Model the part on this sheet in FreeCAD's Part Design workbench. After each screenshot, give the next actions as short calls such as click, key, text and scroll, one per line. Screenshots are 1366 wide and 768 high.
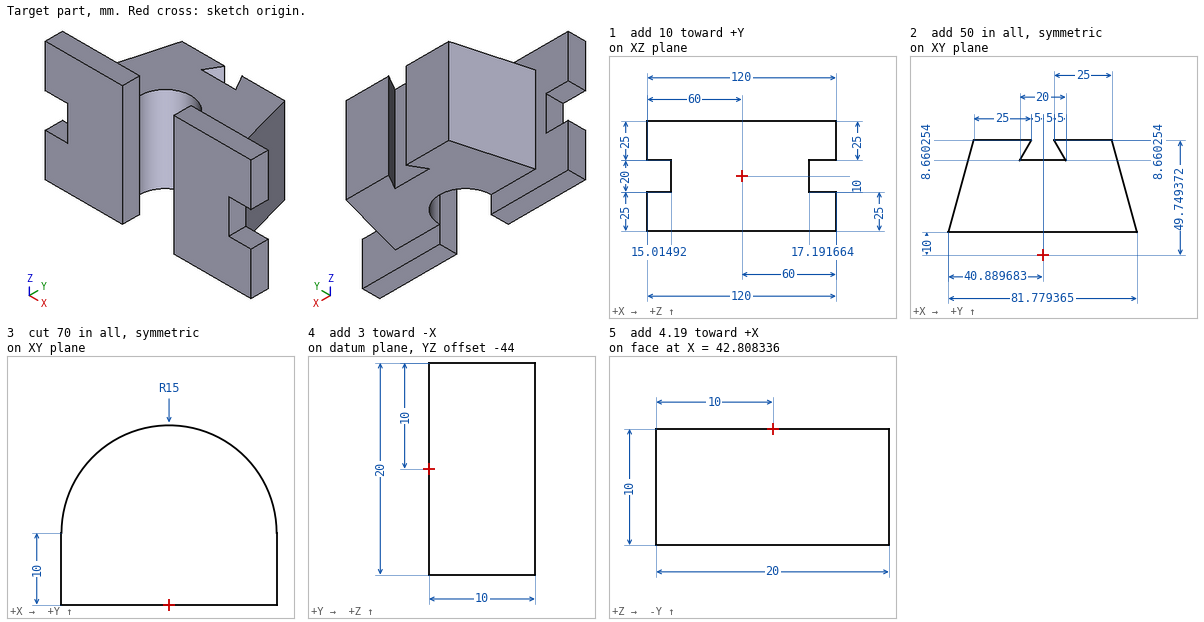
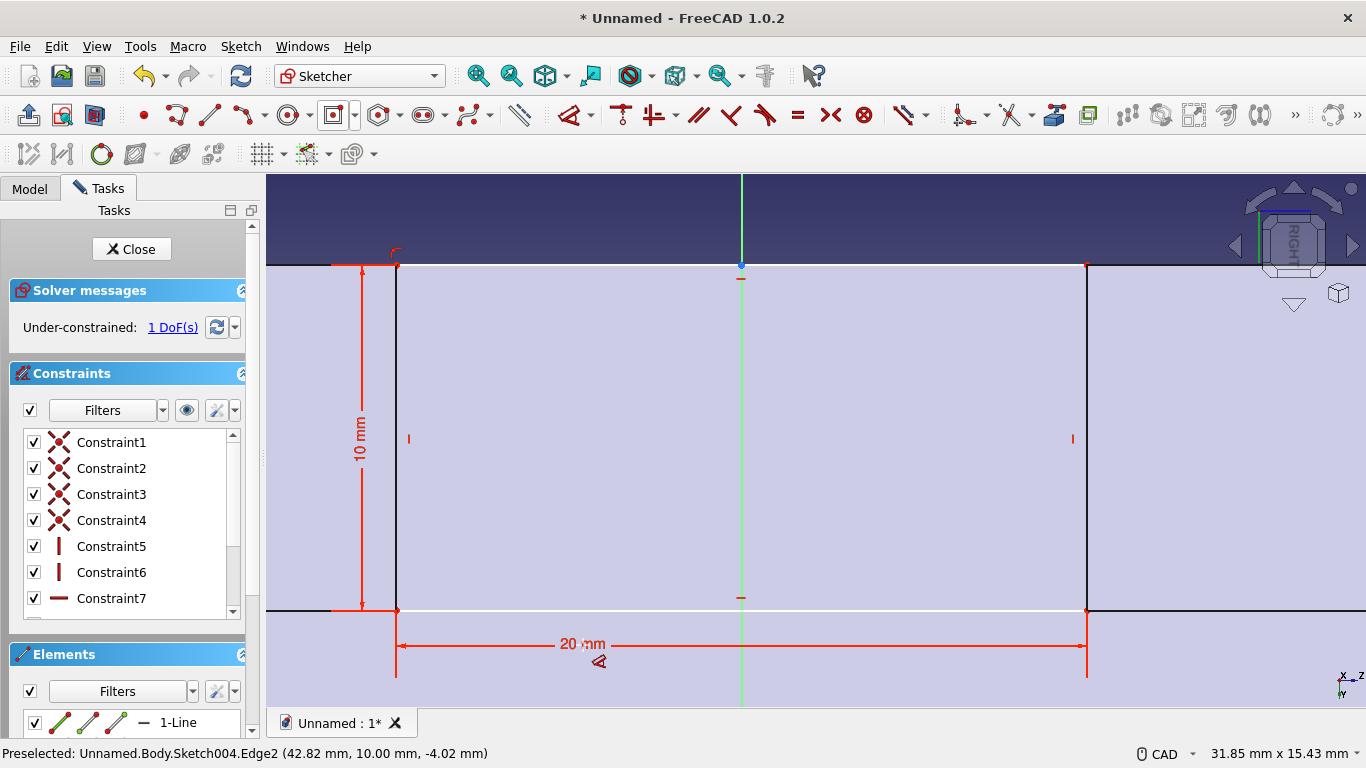
click(396, 265)
click(569, 231)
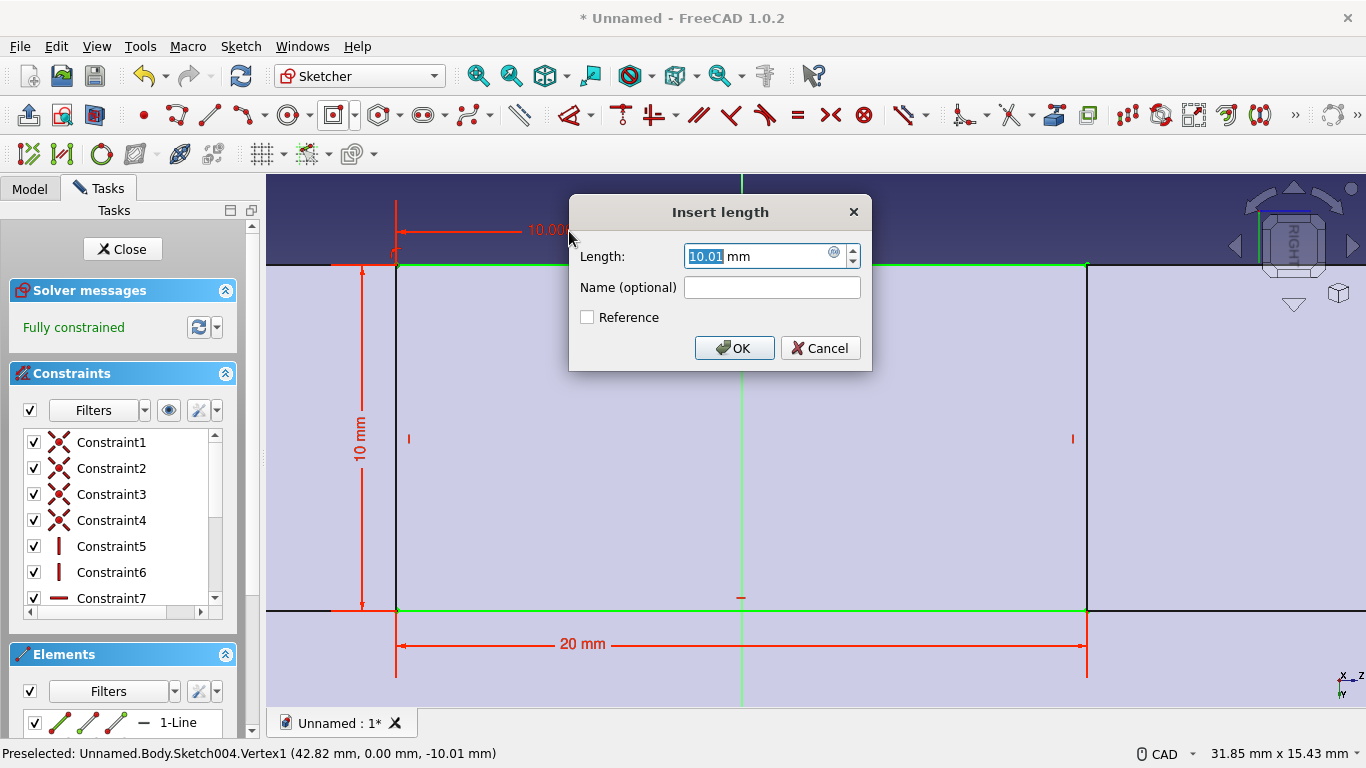
text(10)
key(Return)
key(Escape)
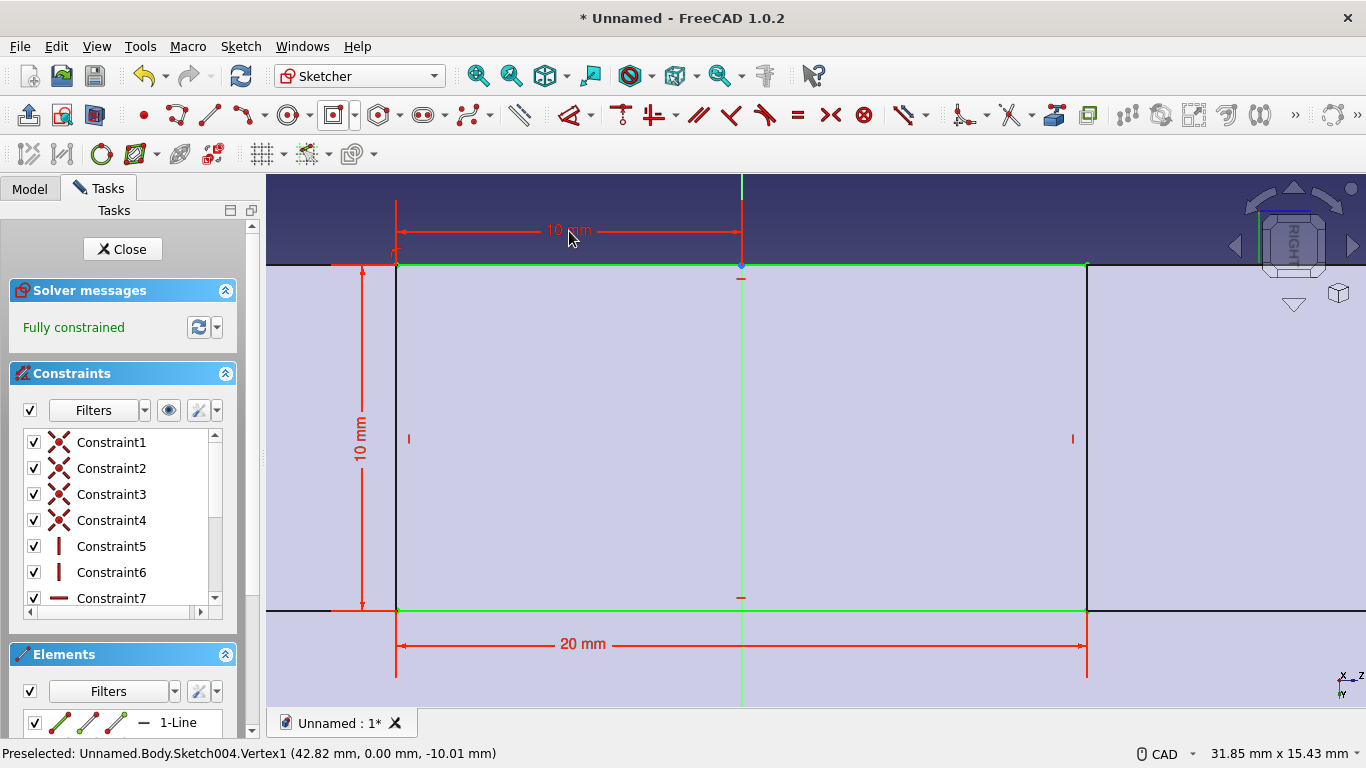
click(123, 249)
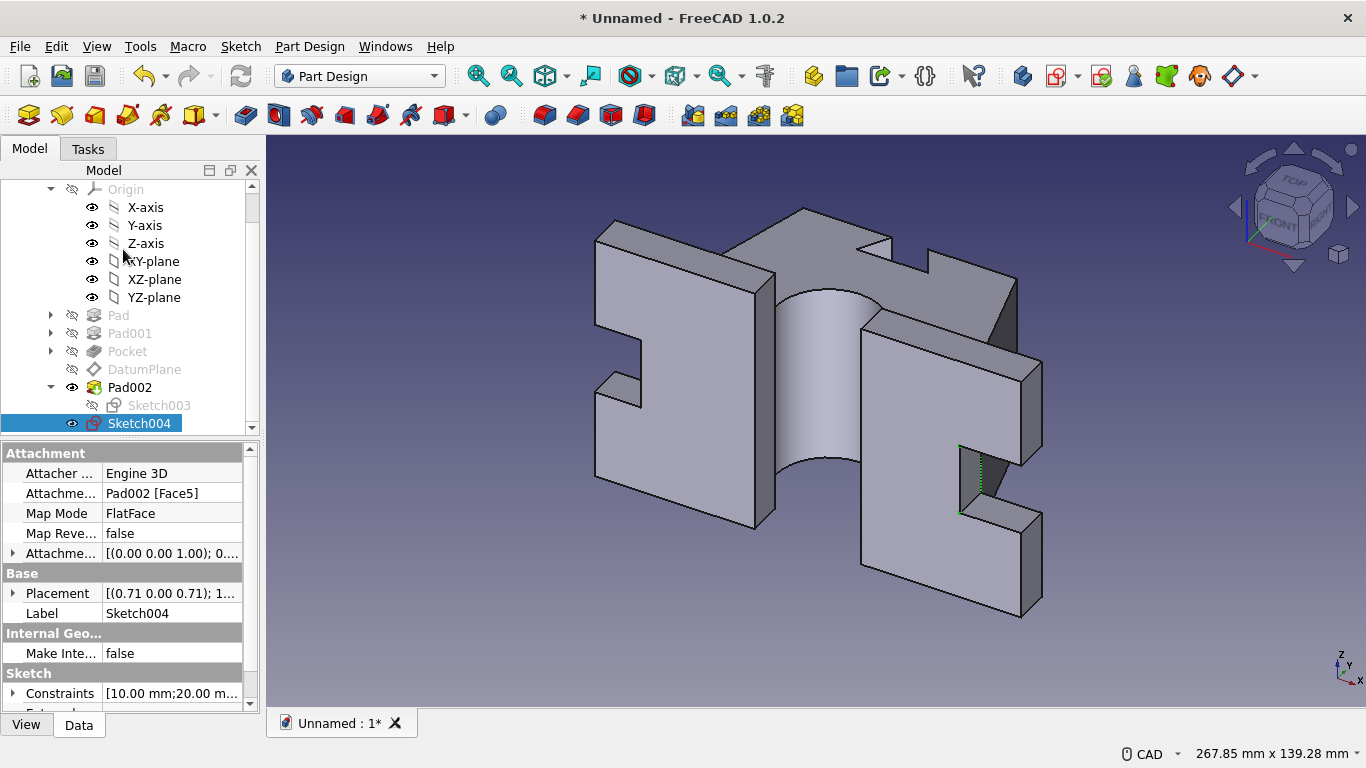
click(29, 116)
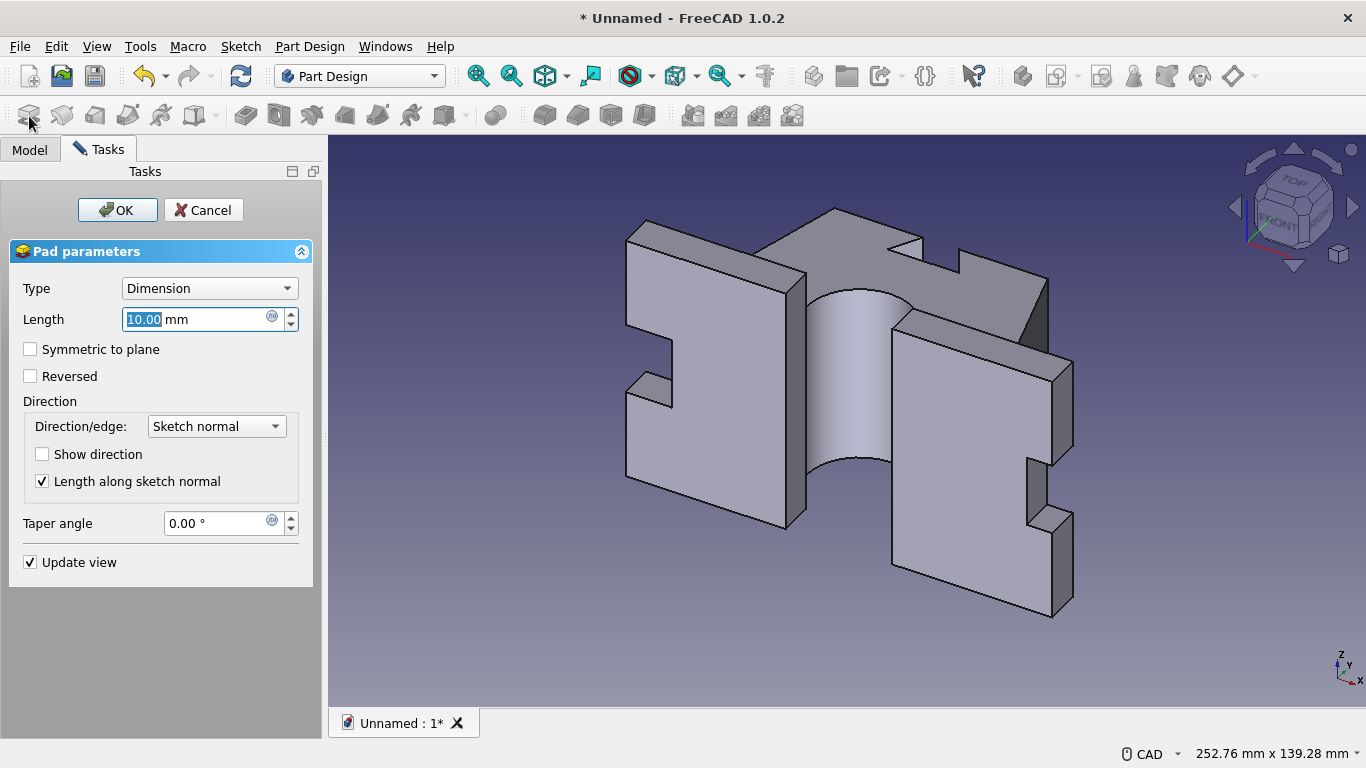
text(4.19)
key(Tab)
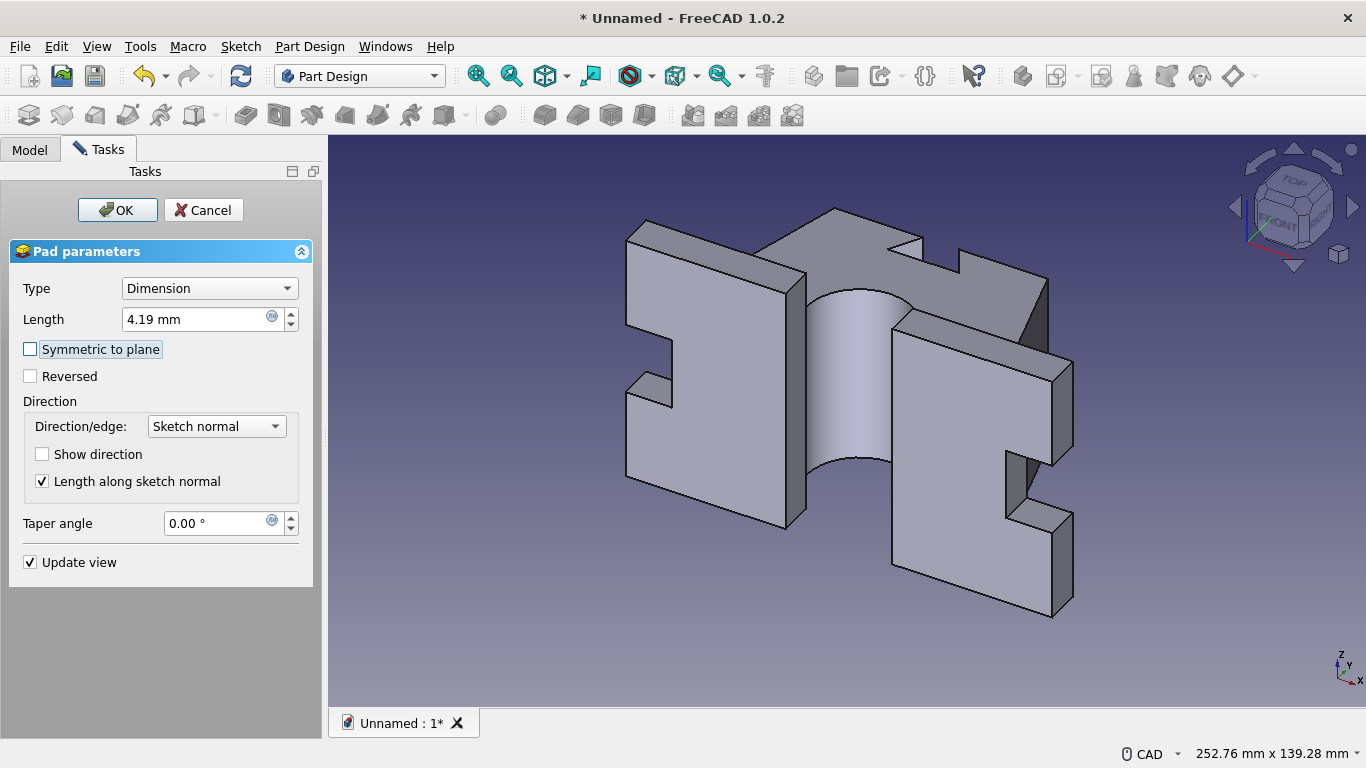
click(118, 210)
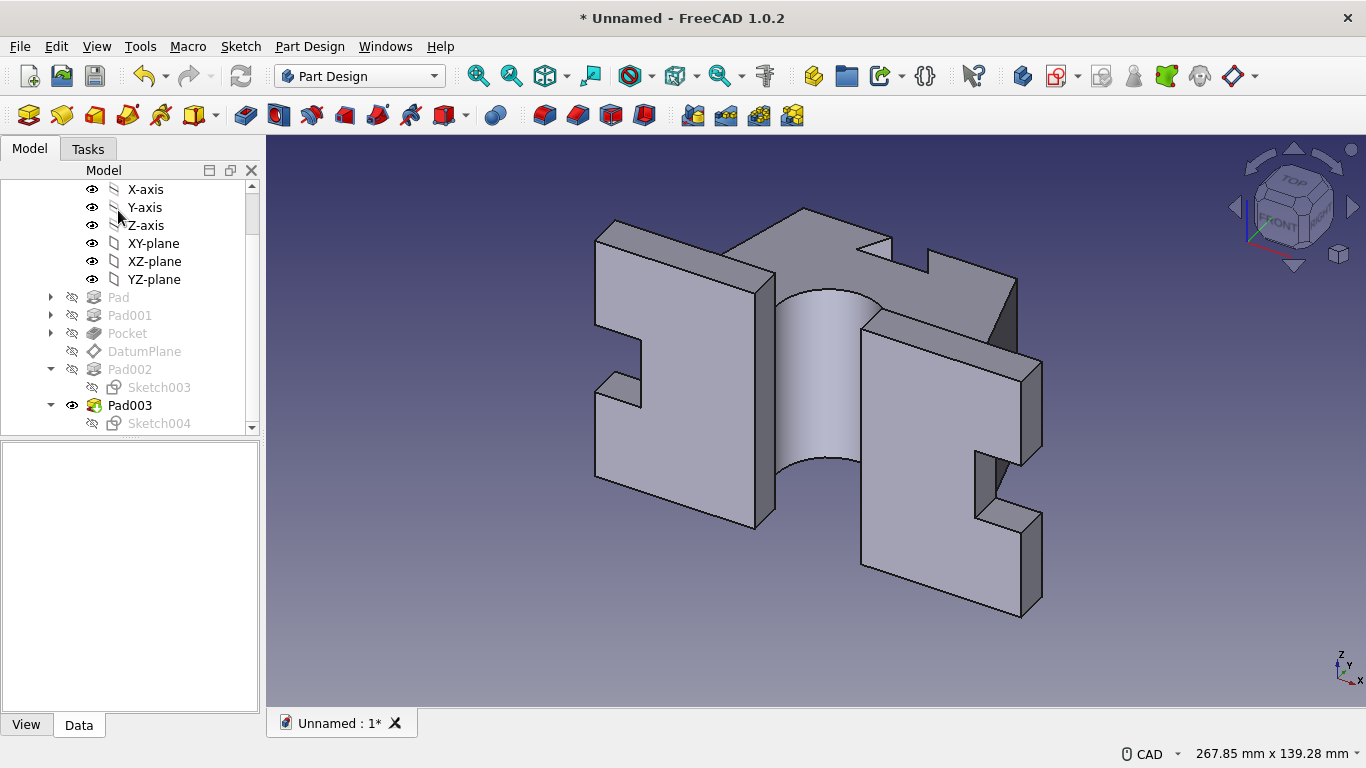
key(0)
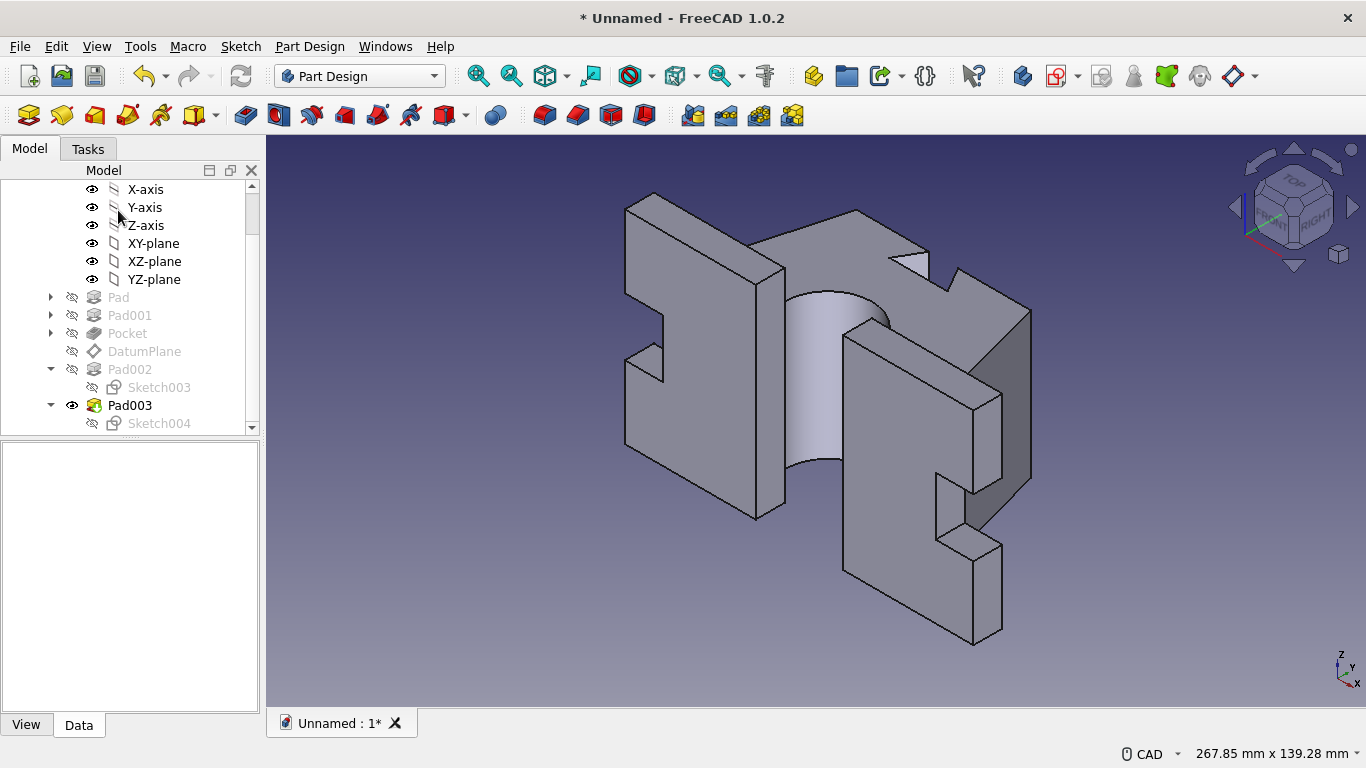
click(479, 76)